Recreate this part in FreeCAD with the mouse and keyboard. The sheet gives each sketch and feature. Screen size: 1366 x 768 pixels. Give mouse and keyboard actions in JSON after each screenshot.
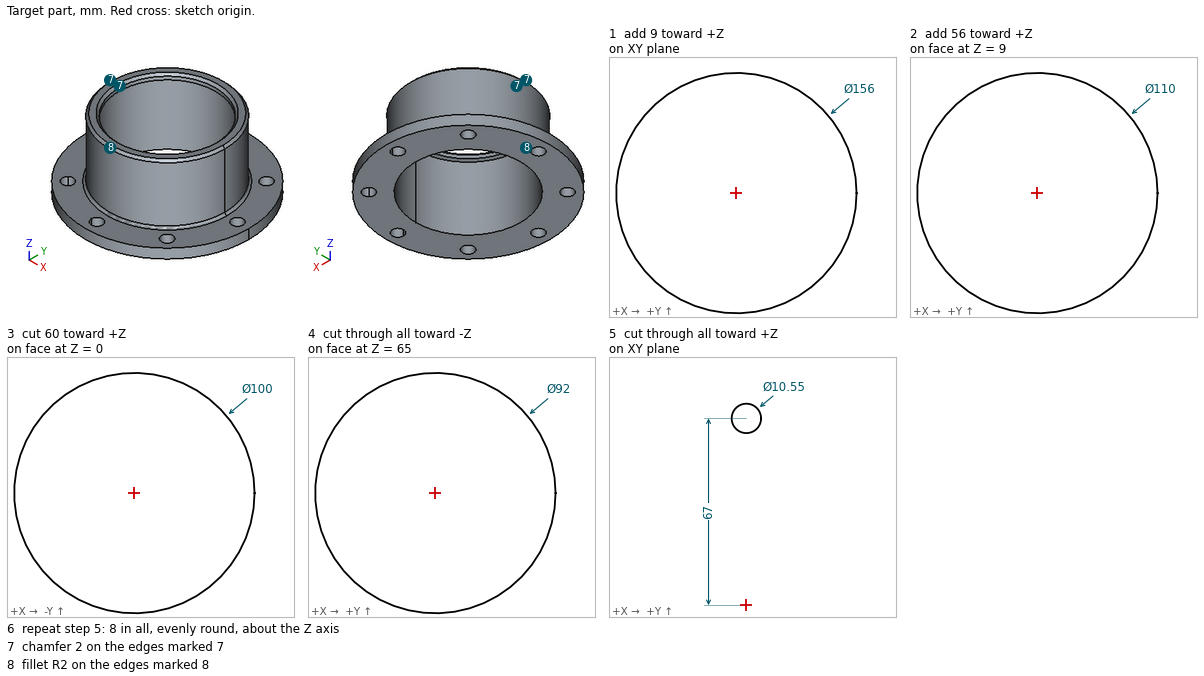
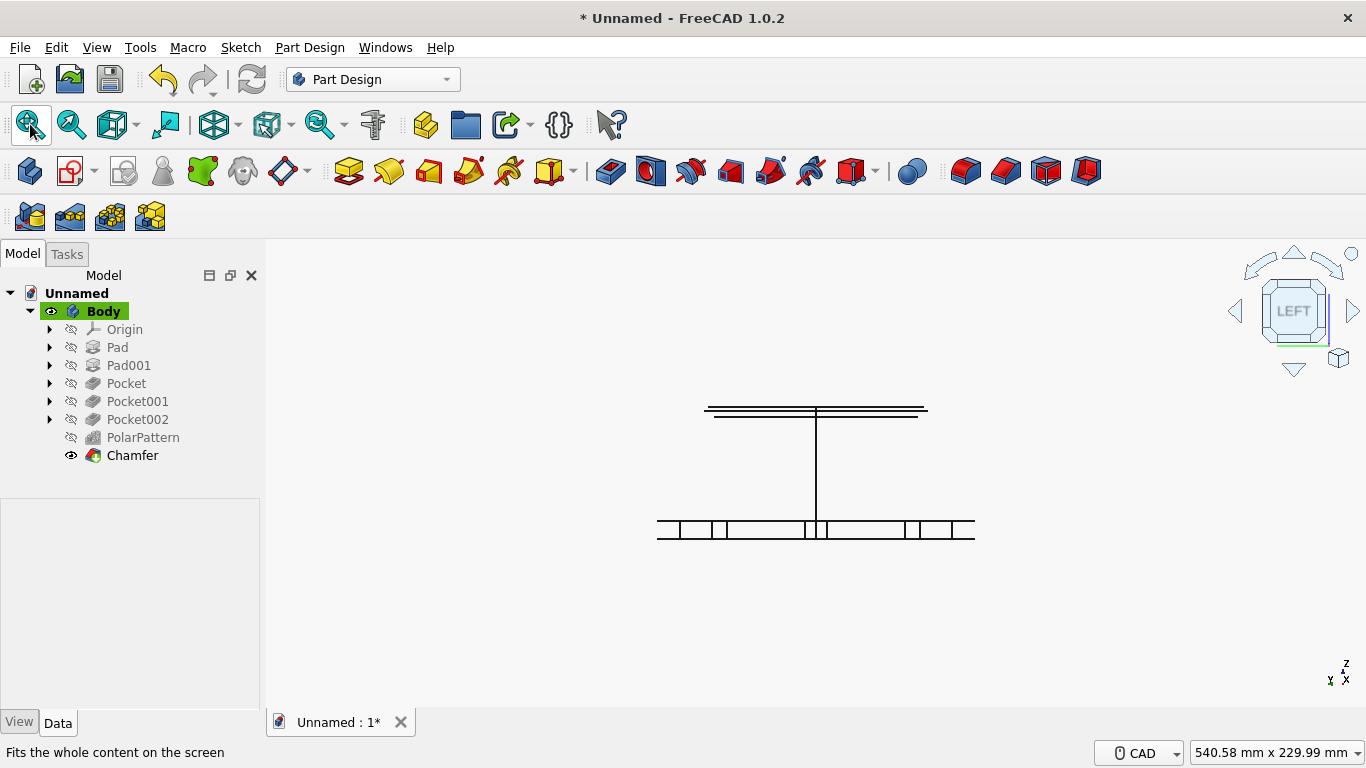
{"action": "key", "text": "0"}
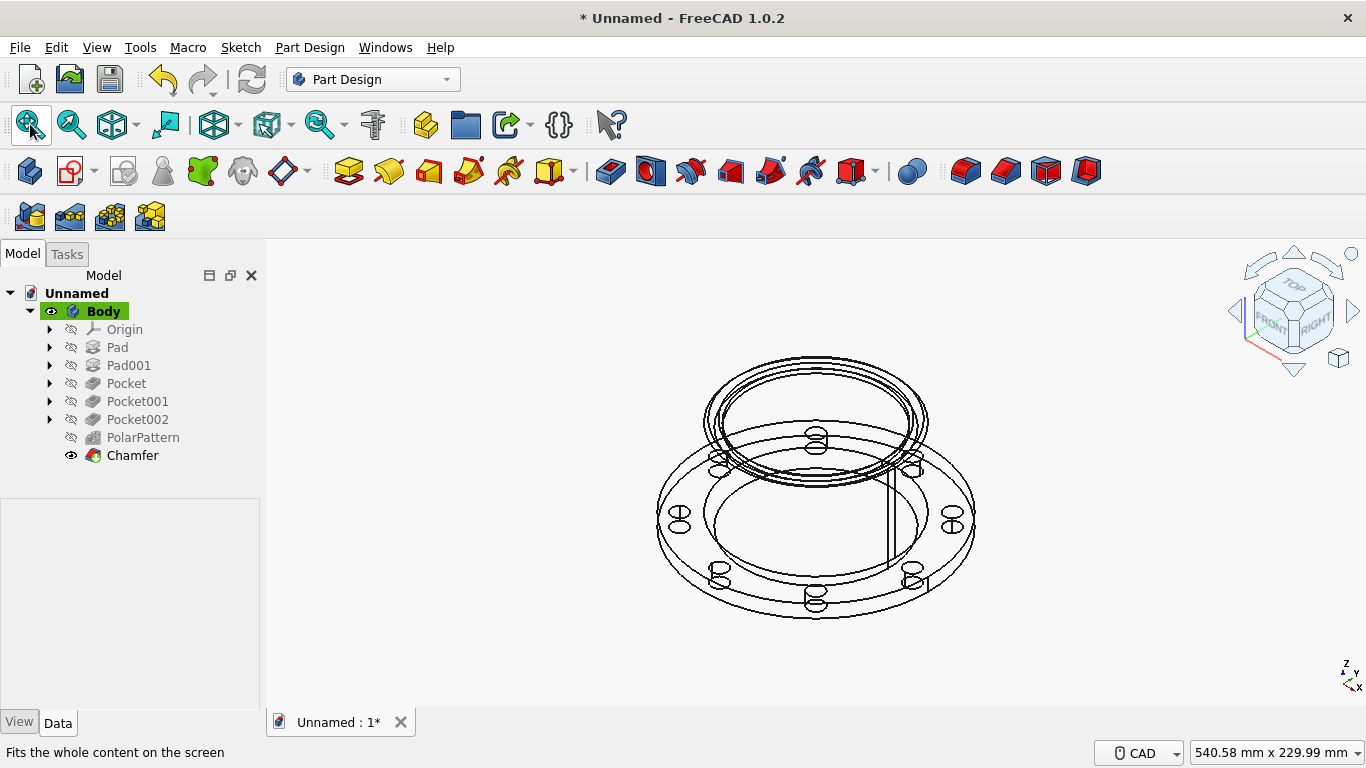
{"action": "left_click", "coordinate": [798, 447]}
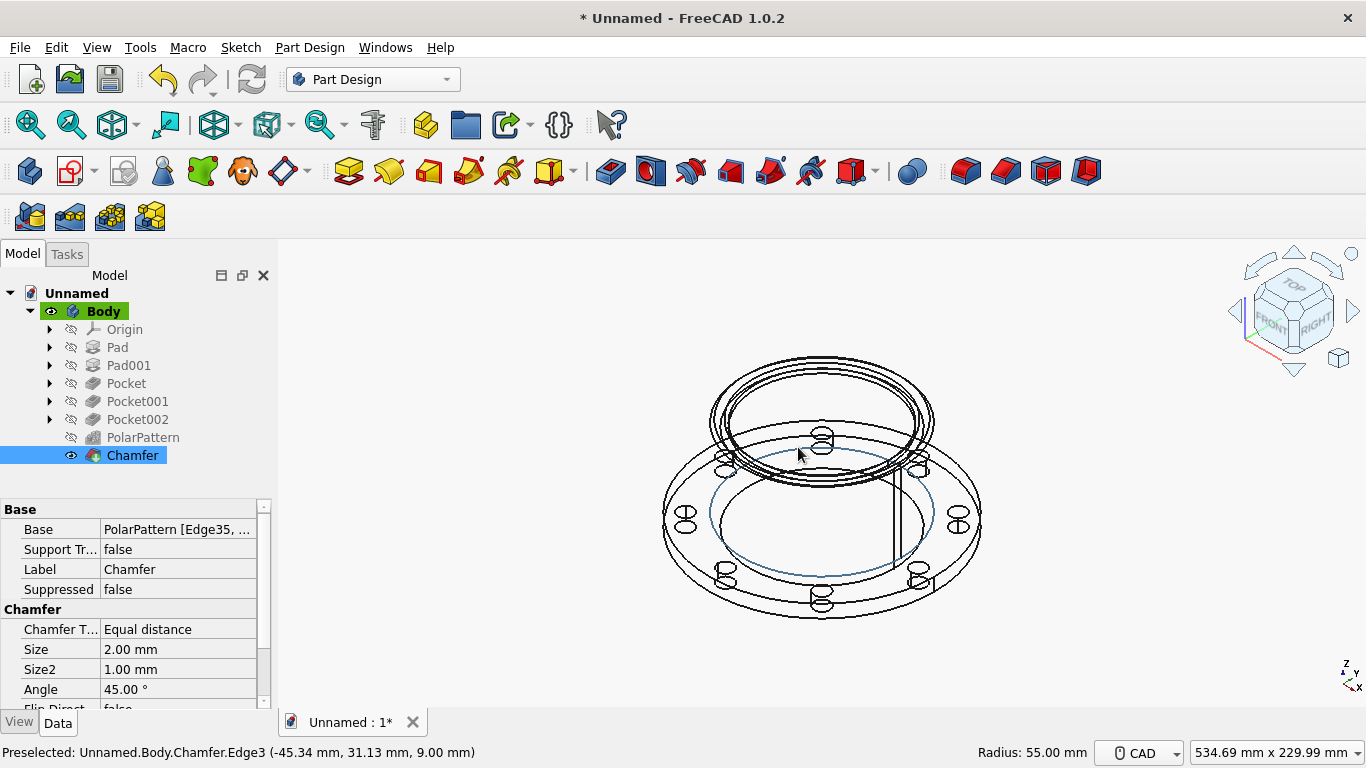
{"action": "key", "text": "v 1"}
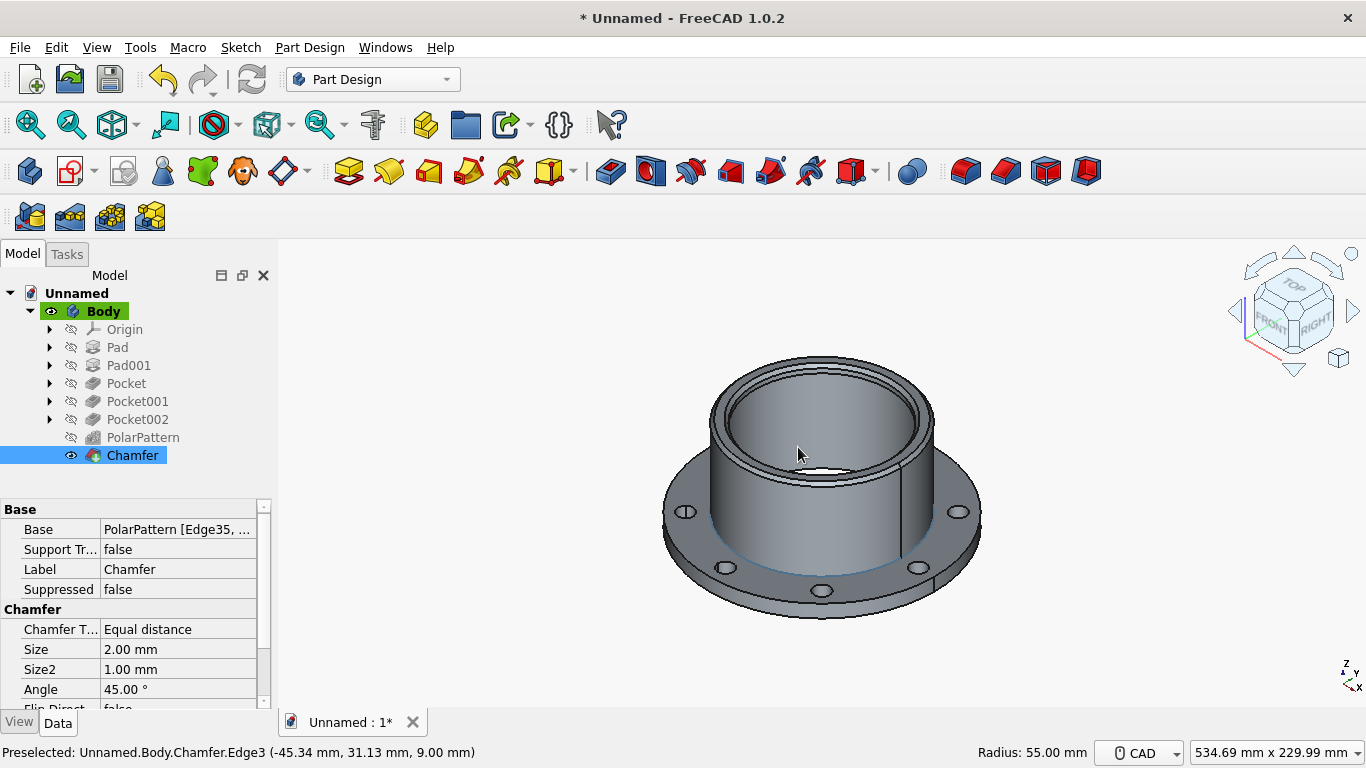
{"action": "left_click", "coordinate": [966, 172]}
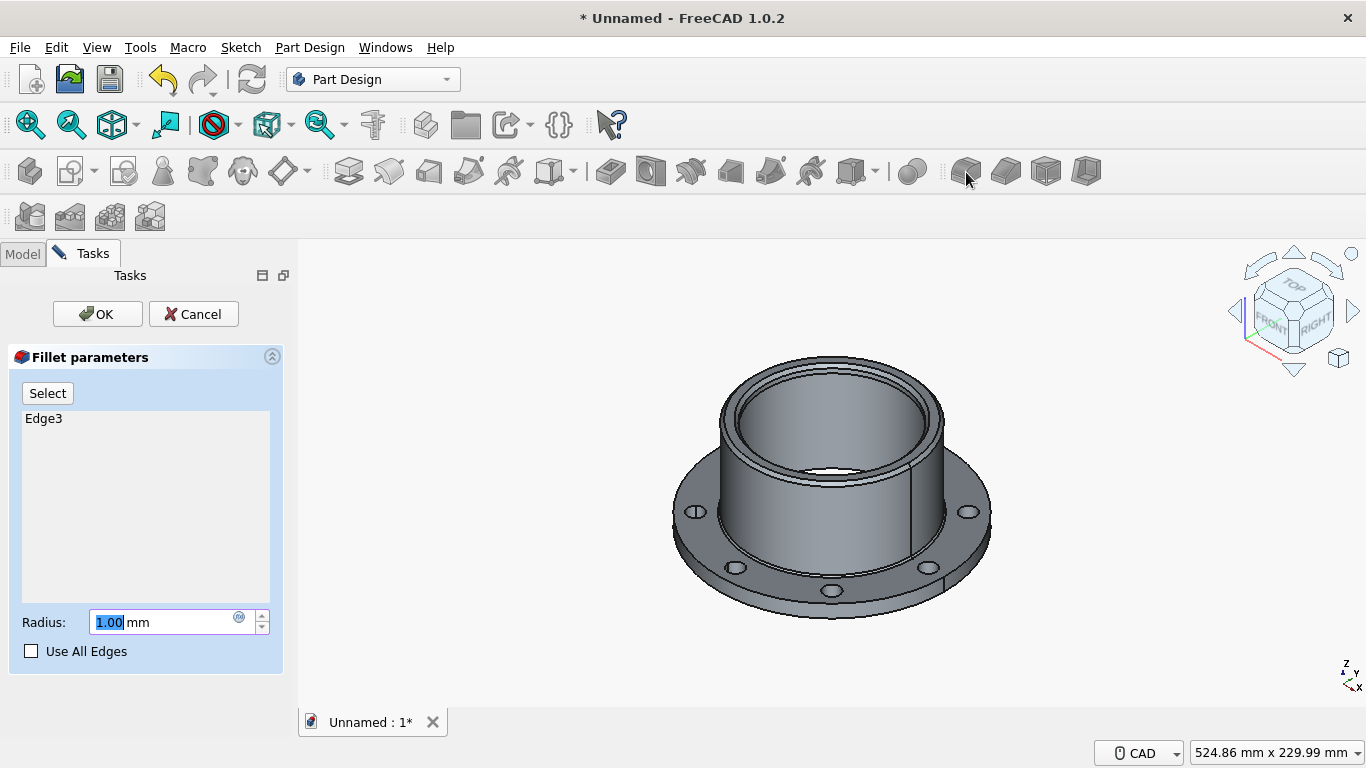
{"action": "type", "text": "2"}
{"action": "key", "text": "Tab"}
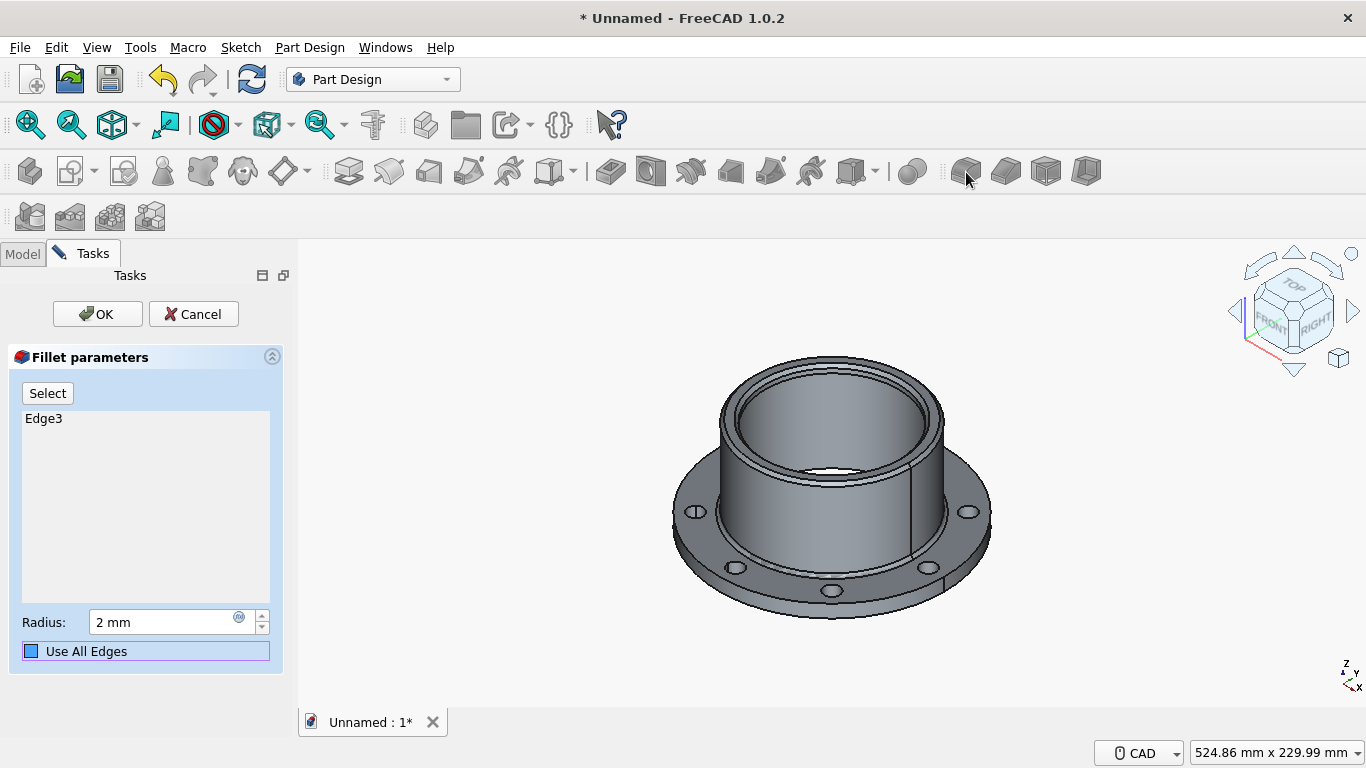
{"action": "left_click", "coordinate": [98, 314]}